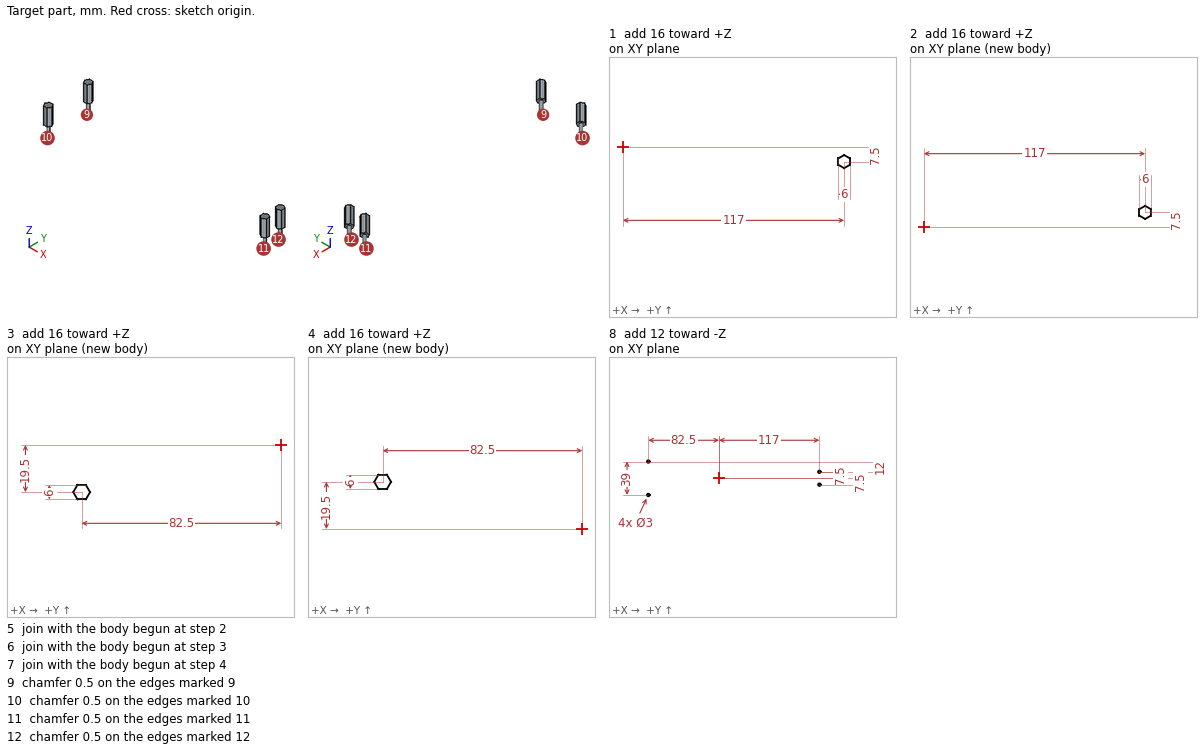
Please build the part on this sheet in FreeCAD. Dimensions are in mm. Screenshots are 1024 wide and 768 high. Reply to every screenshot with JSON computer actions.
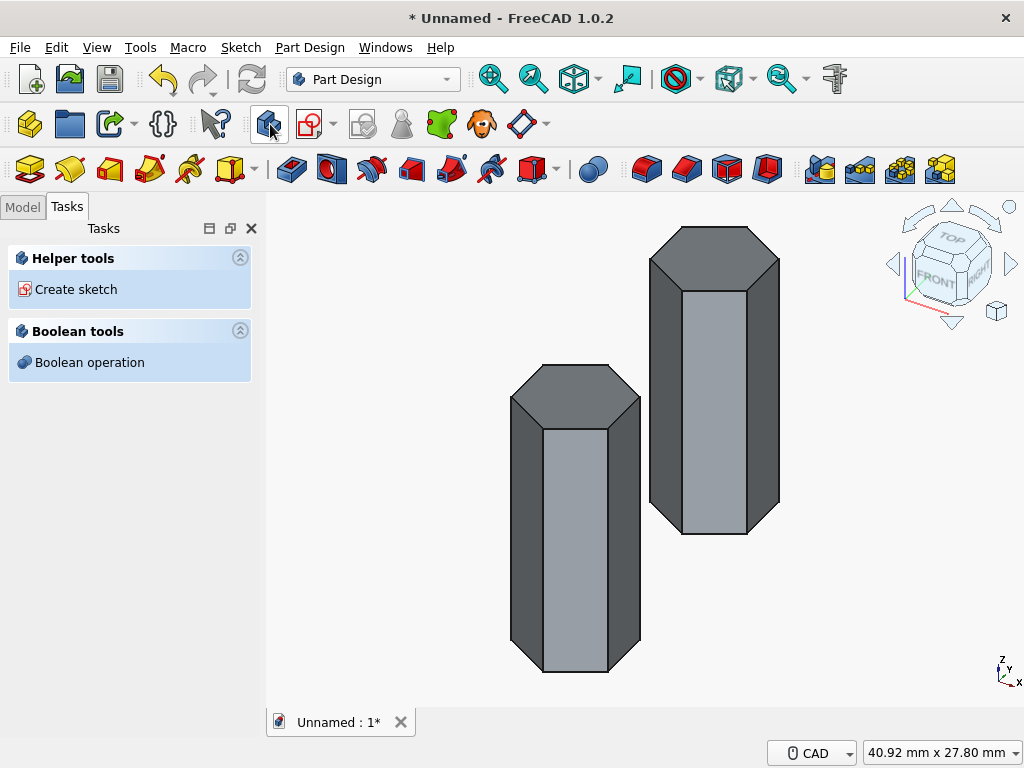
{"action": "left_click", "coordinate": [306, 667]}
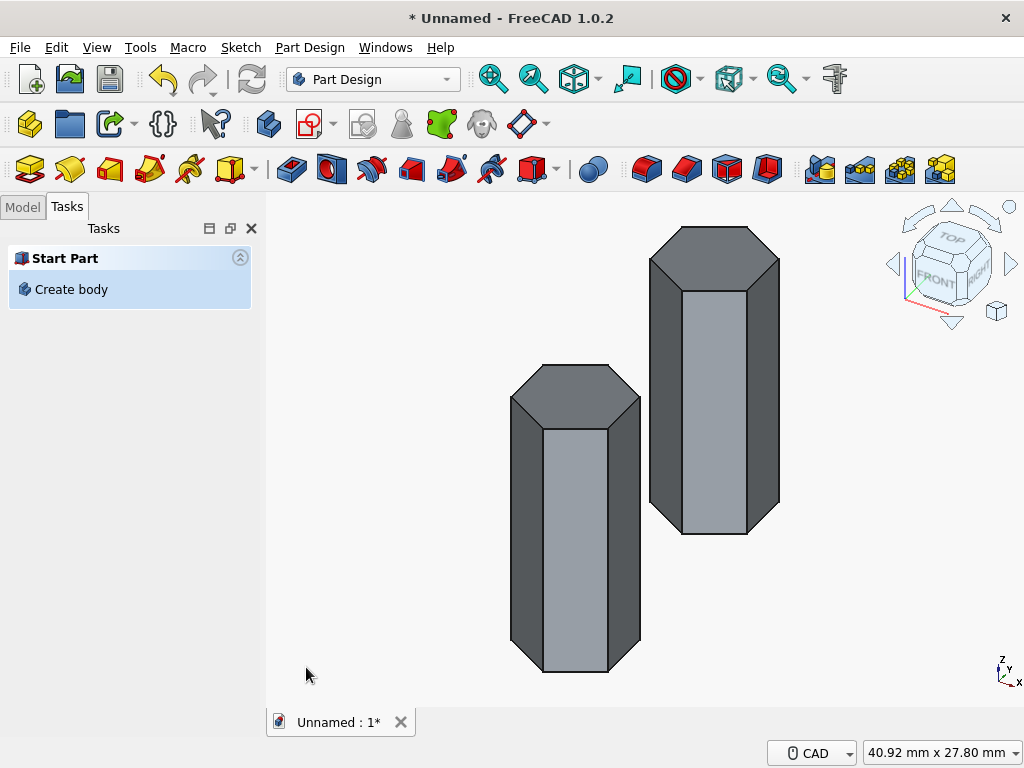
{"action": "left_click", "coordinate": [310, 124]}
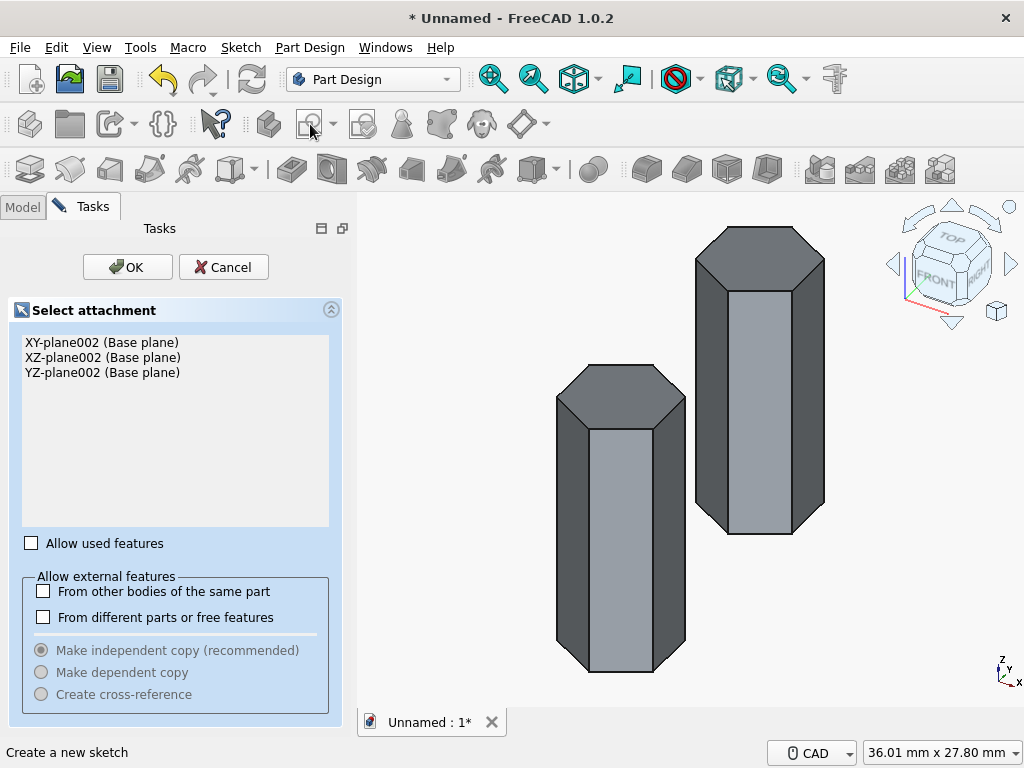
{"action": "left_click", "coordinate": [82, 342]}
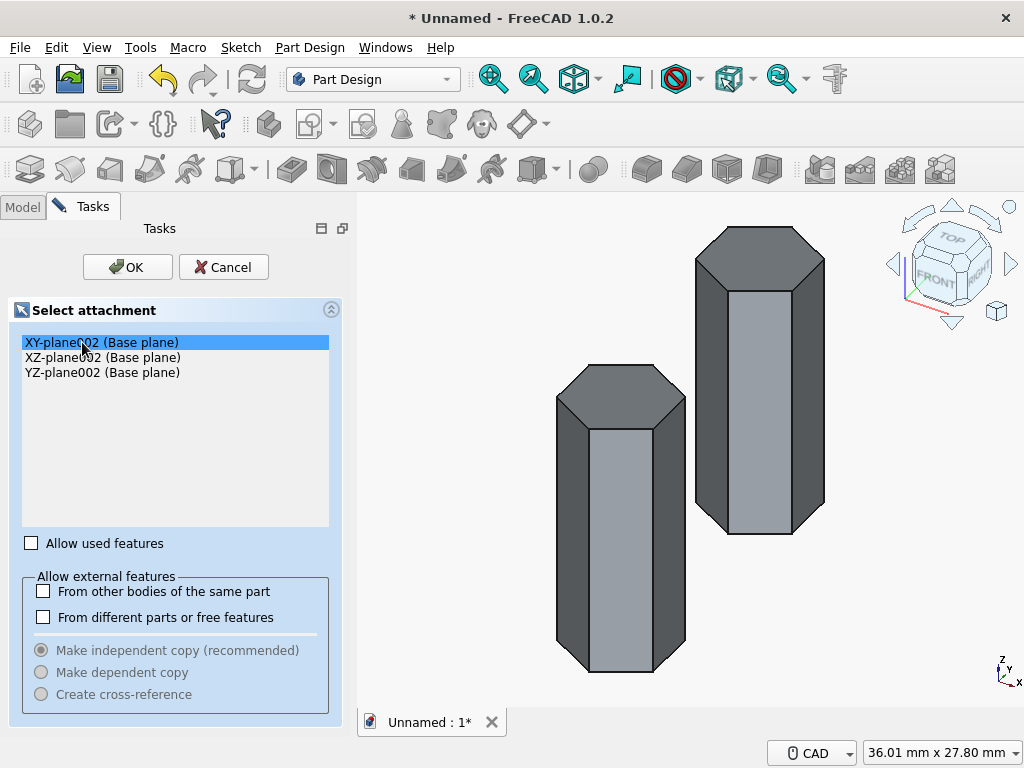
{"action": "left_click", "coordinate": [128, 267]}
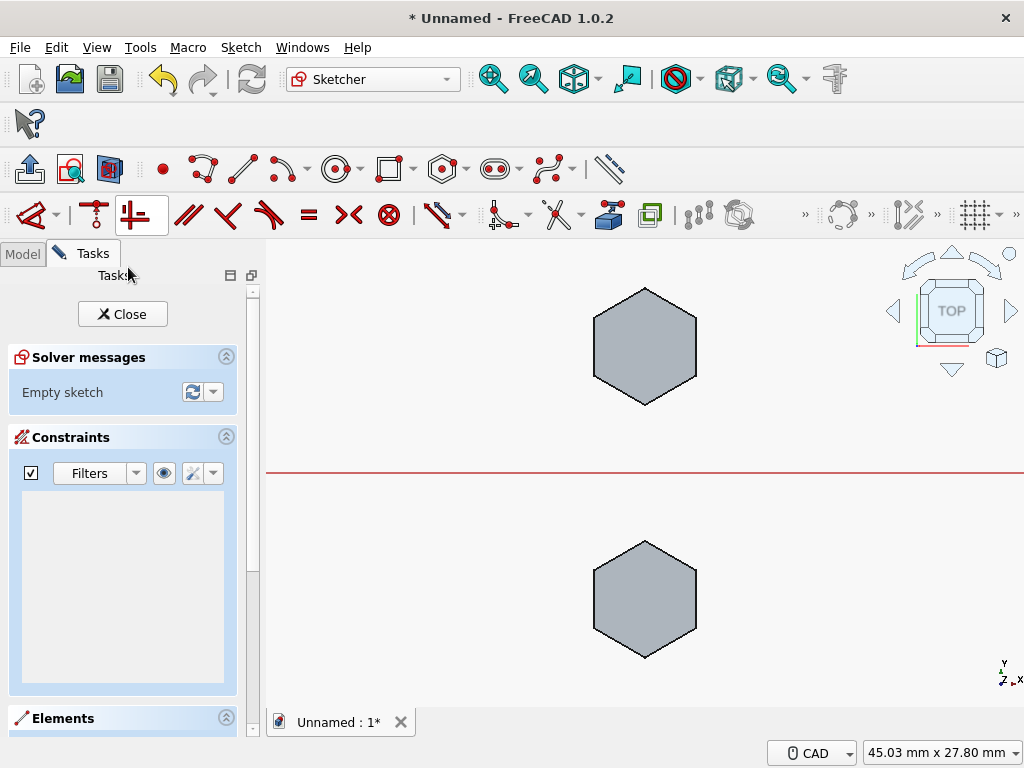
{"action": "scroll", "coordinate": [576, 473], "scroll_direction": "down", "scroll_amount": 5}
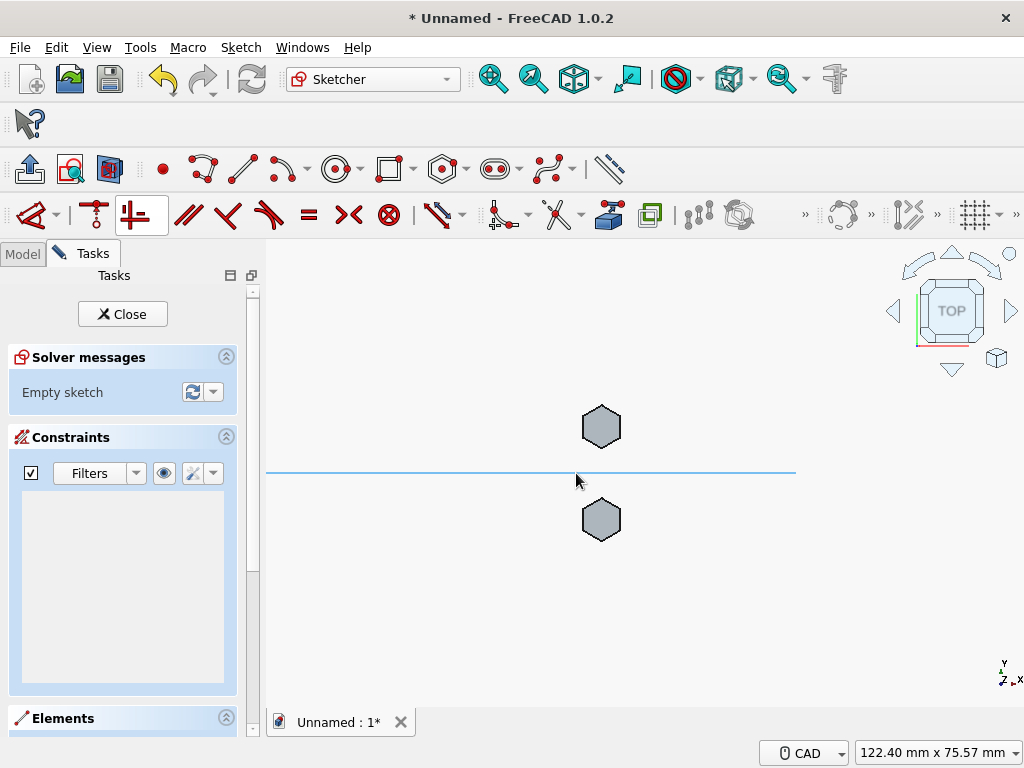
{"action": "scroll", "coordinate": [576, 473], "scroll_direction": "down", "scroll_amount": 5}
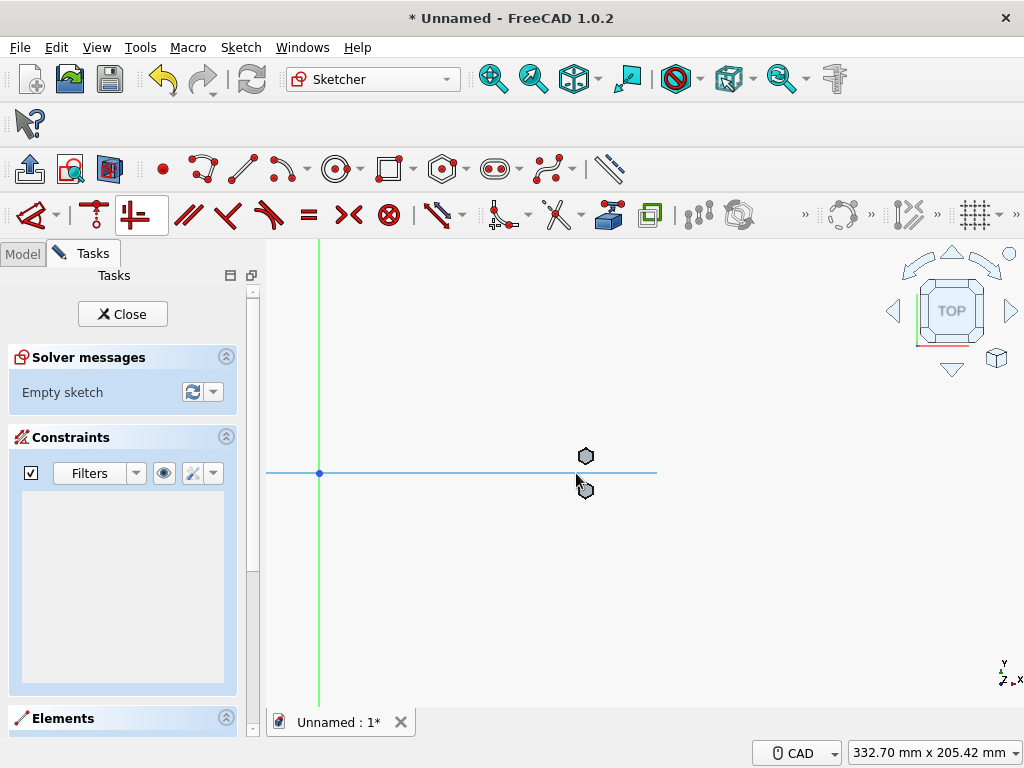
{"action": "scroll", "coordinate": [576, 473], "scroll_direction": "down", "scroll_amount": 5}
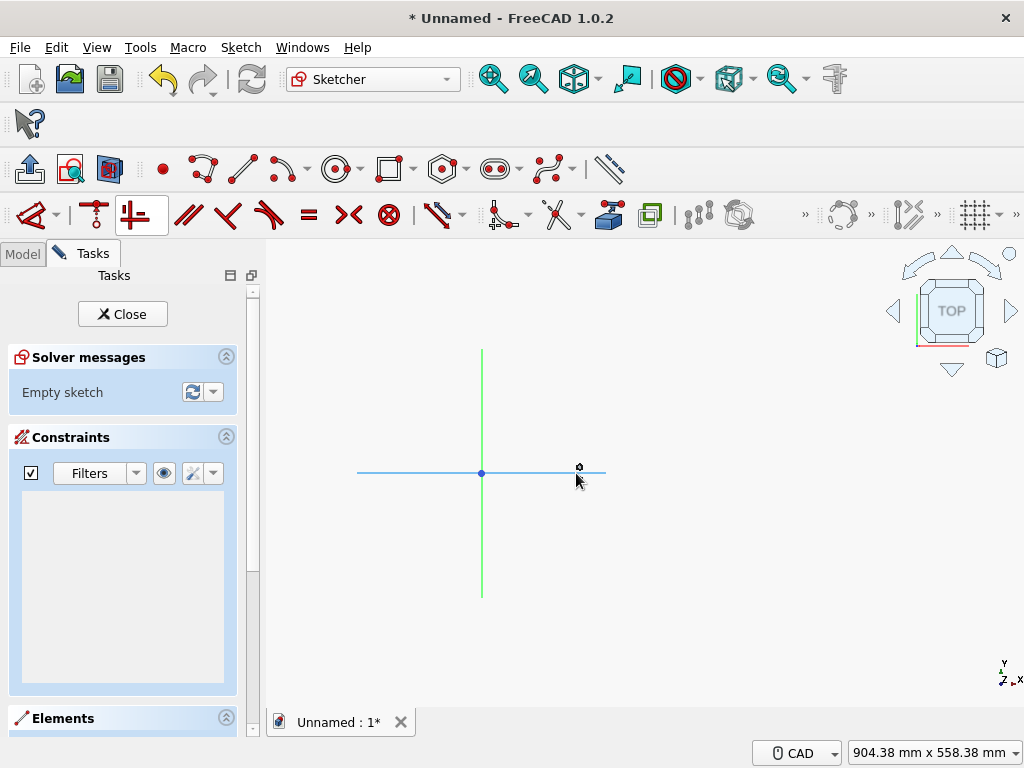
{"action": "scroll", "coordinate": [404, 491], "scroll_direction": "up", "scroll_amount": 15}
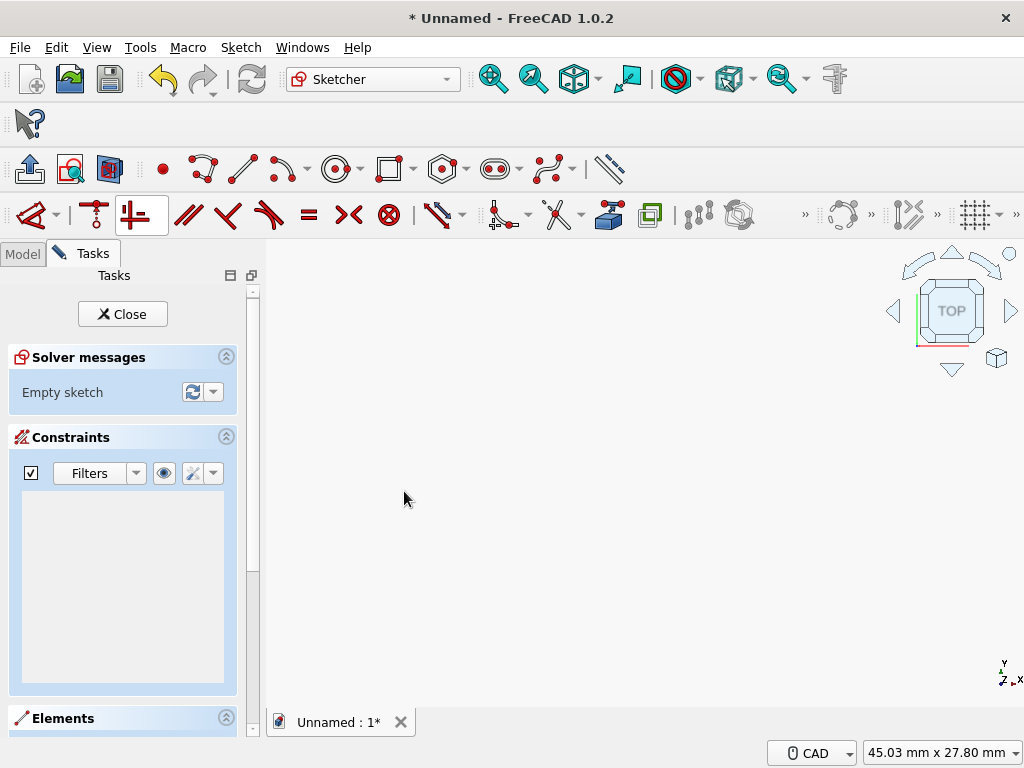
{"action": "scroll", "coordinate": [572, 448], "scroll_direction": "up", "scroll_amount": 5}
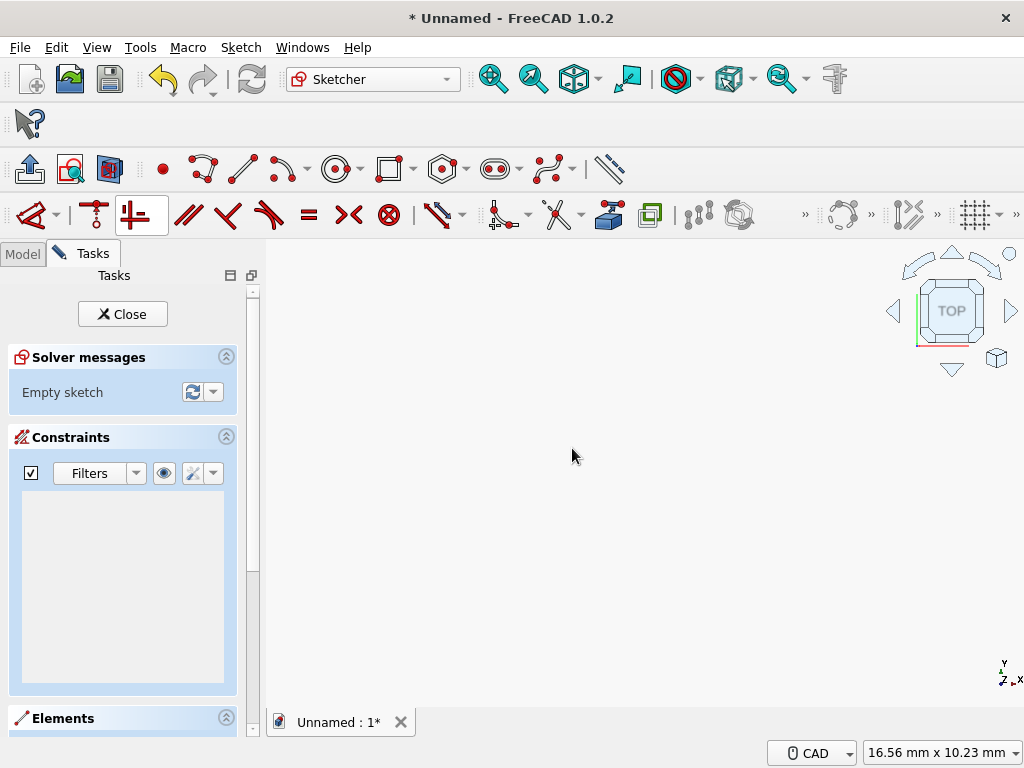
{"action": "left_click", "coordinate": [442, 170]}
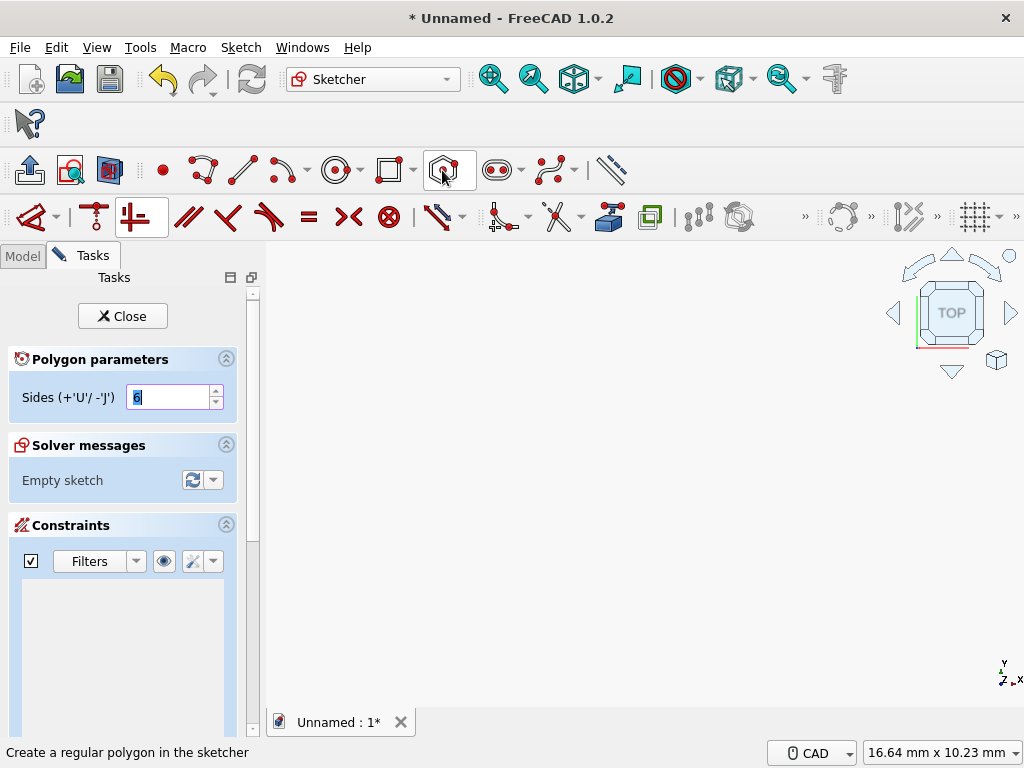
{"action": "left_click", "coordinate": [576, 473]}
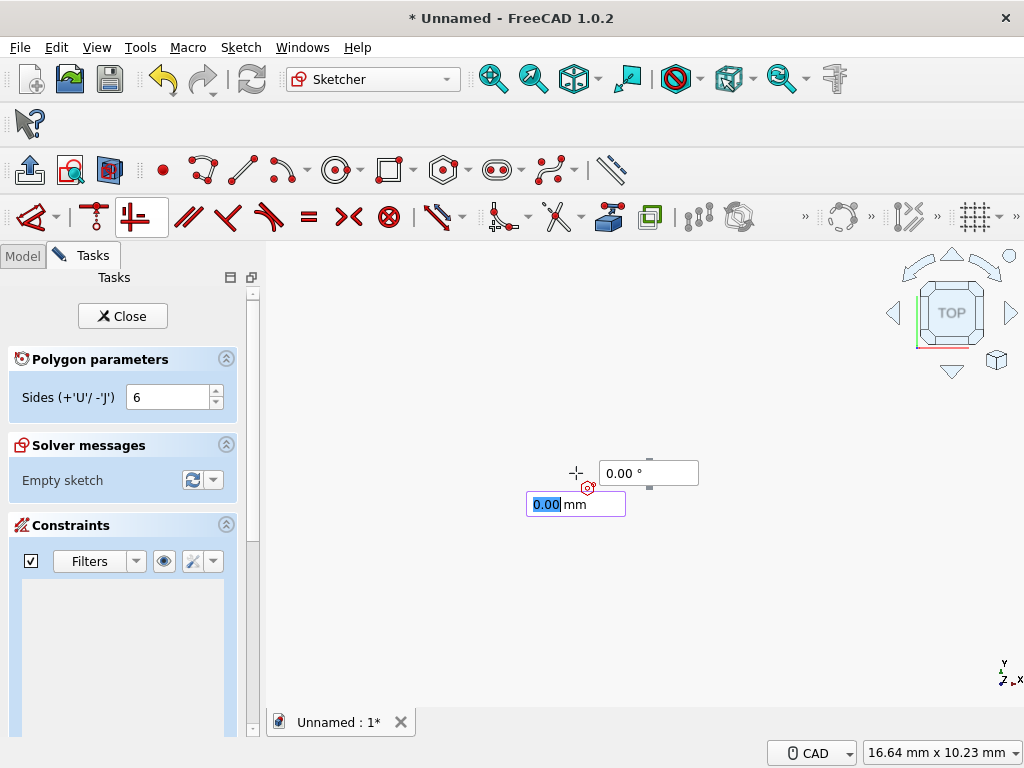
{"action": "left_click", "coordinate": [734, 473]}
{"action": "right_click", "coordinate": [734, 473]}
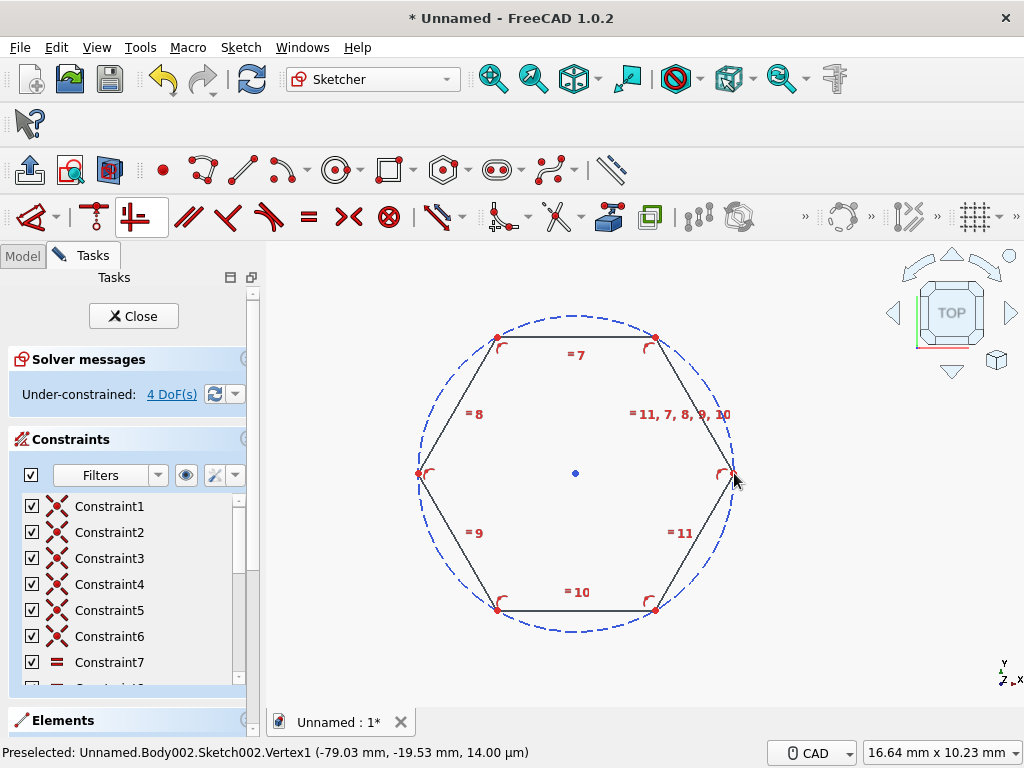
{"action": "left_click", "coordinate": [608, 337]}